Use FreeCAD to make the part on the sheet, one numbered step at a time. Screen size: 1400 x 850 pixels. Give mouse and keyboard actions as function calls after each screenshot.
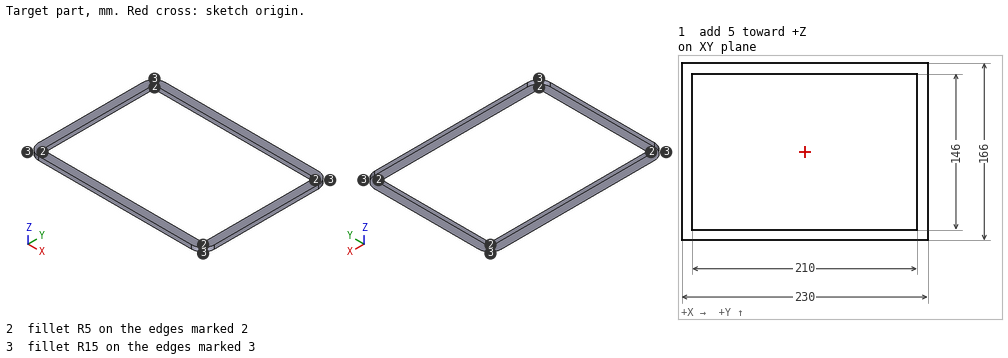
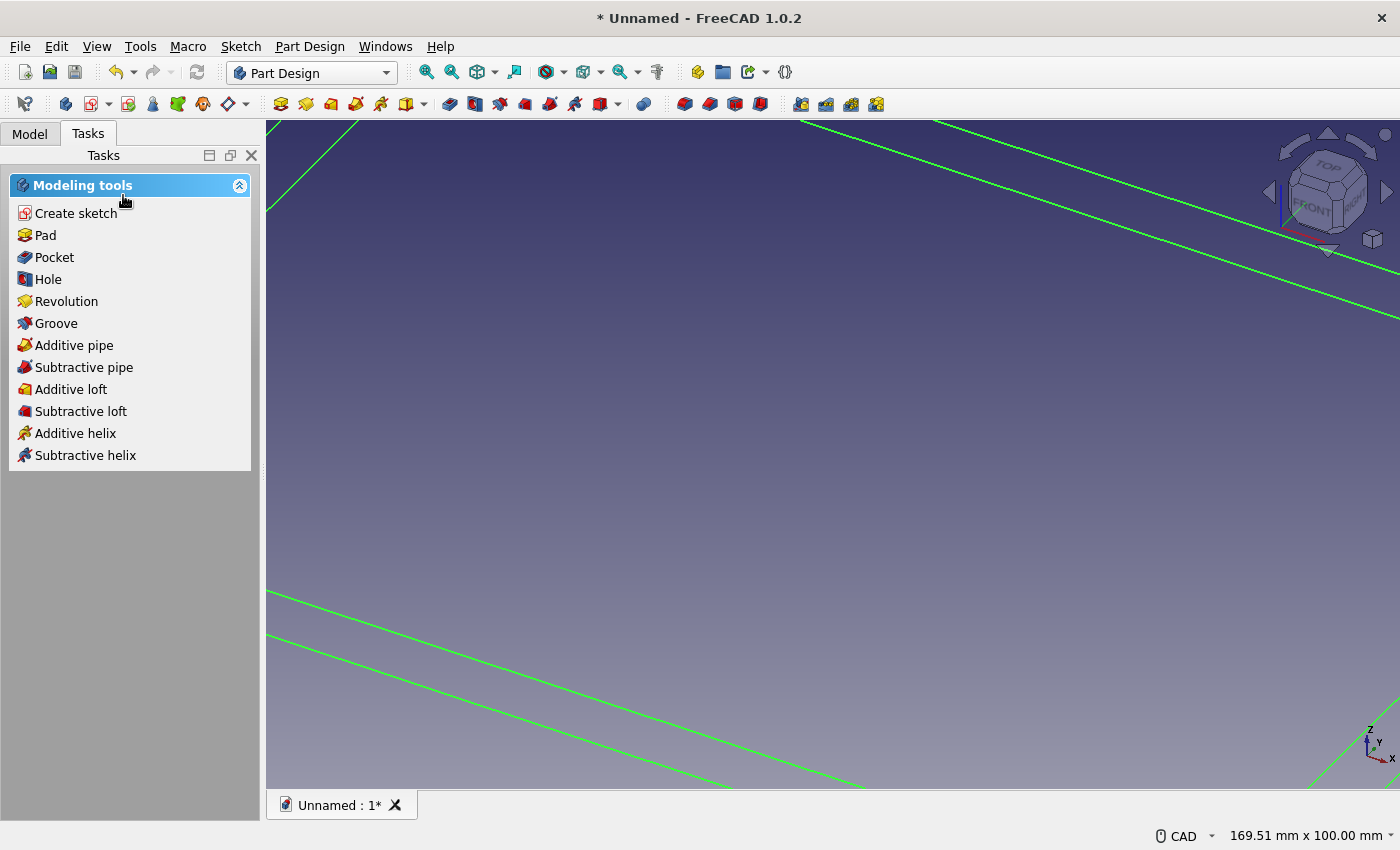
click(281, 104)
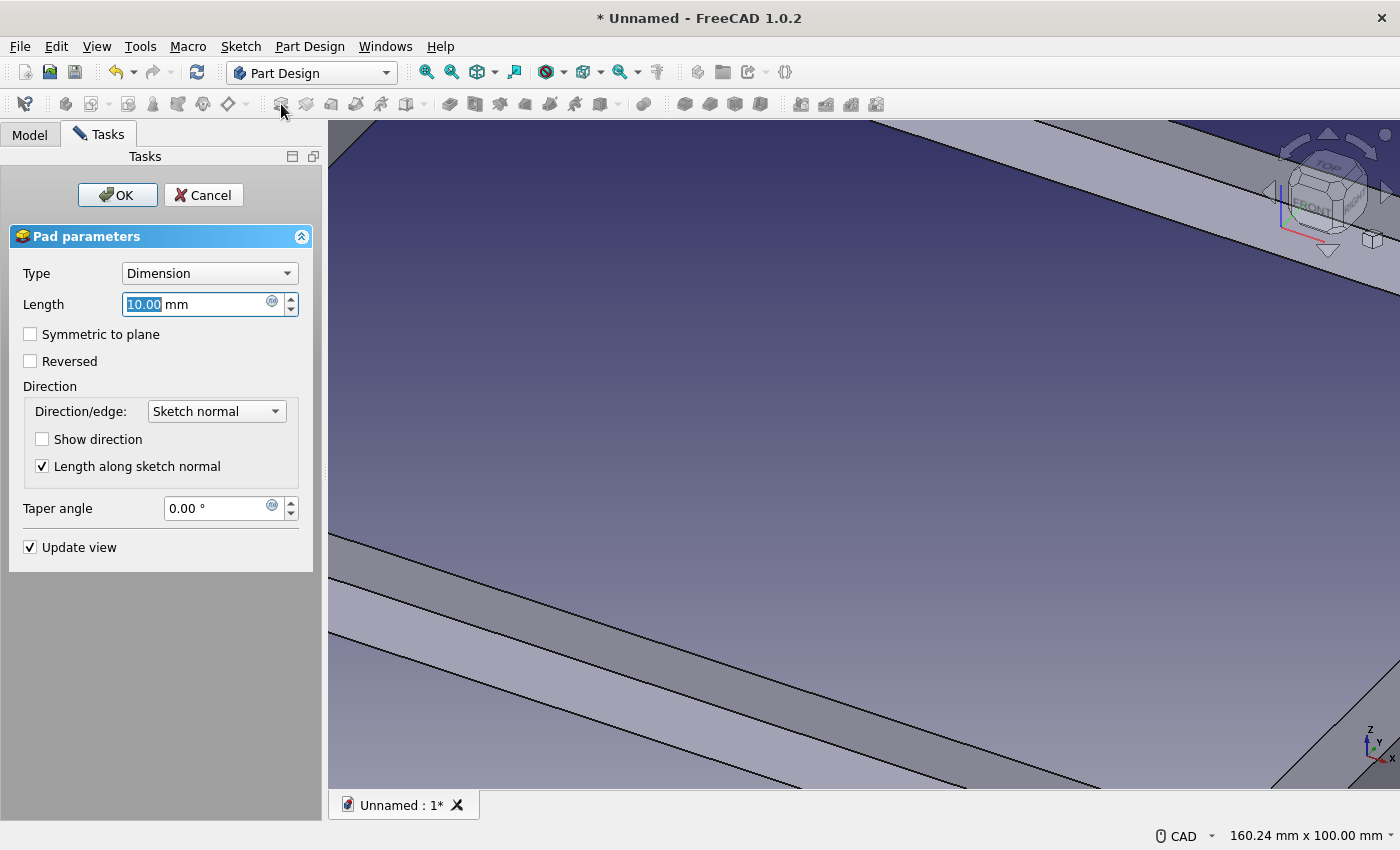
text(5)
key(Tab)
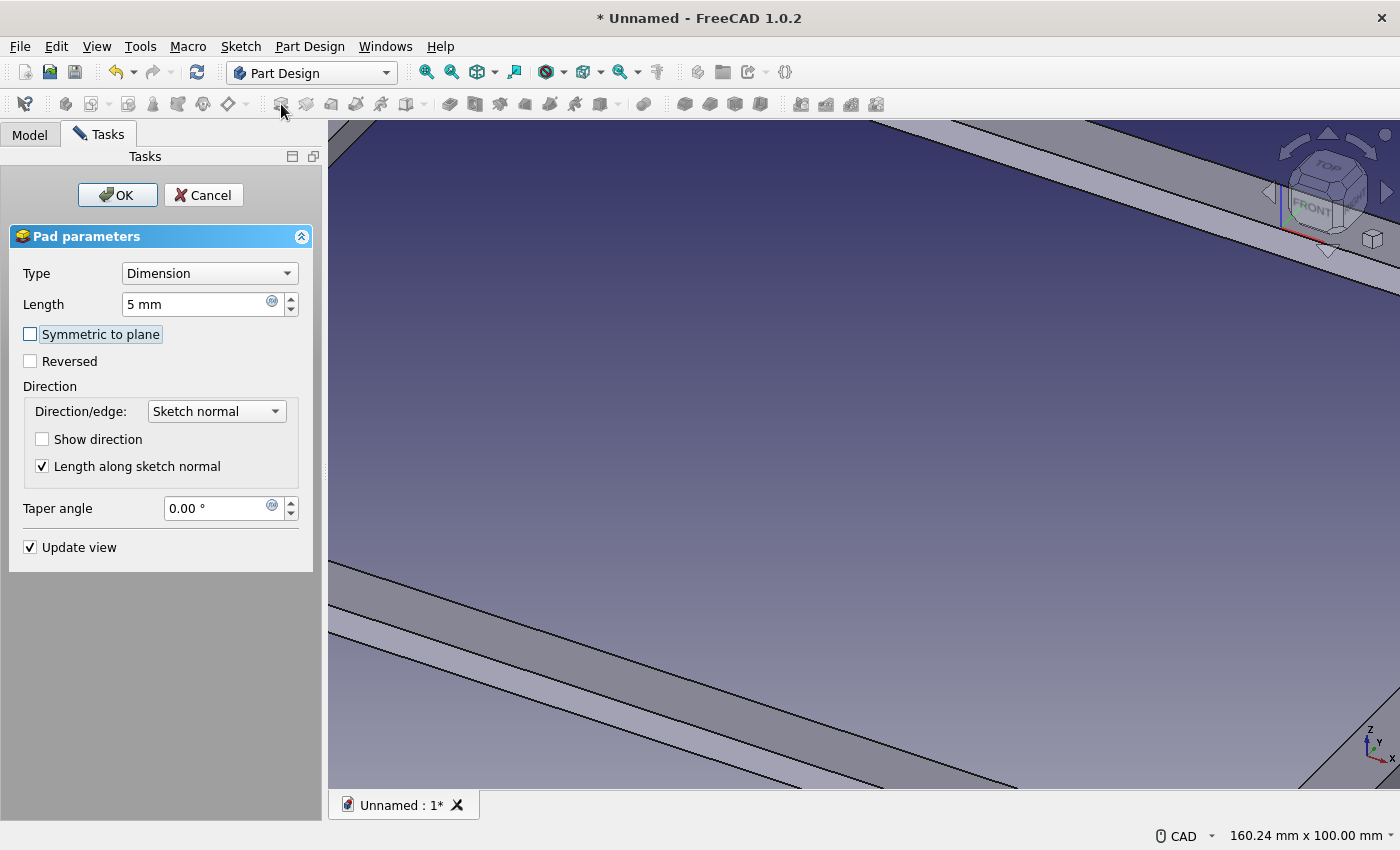
click(118, 195)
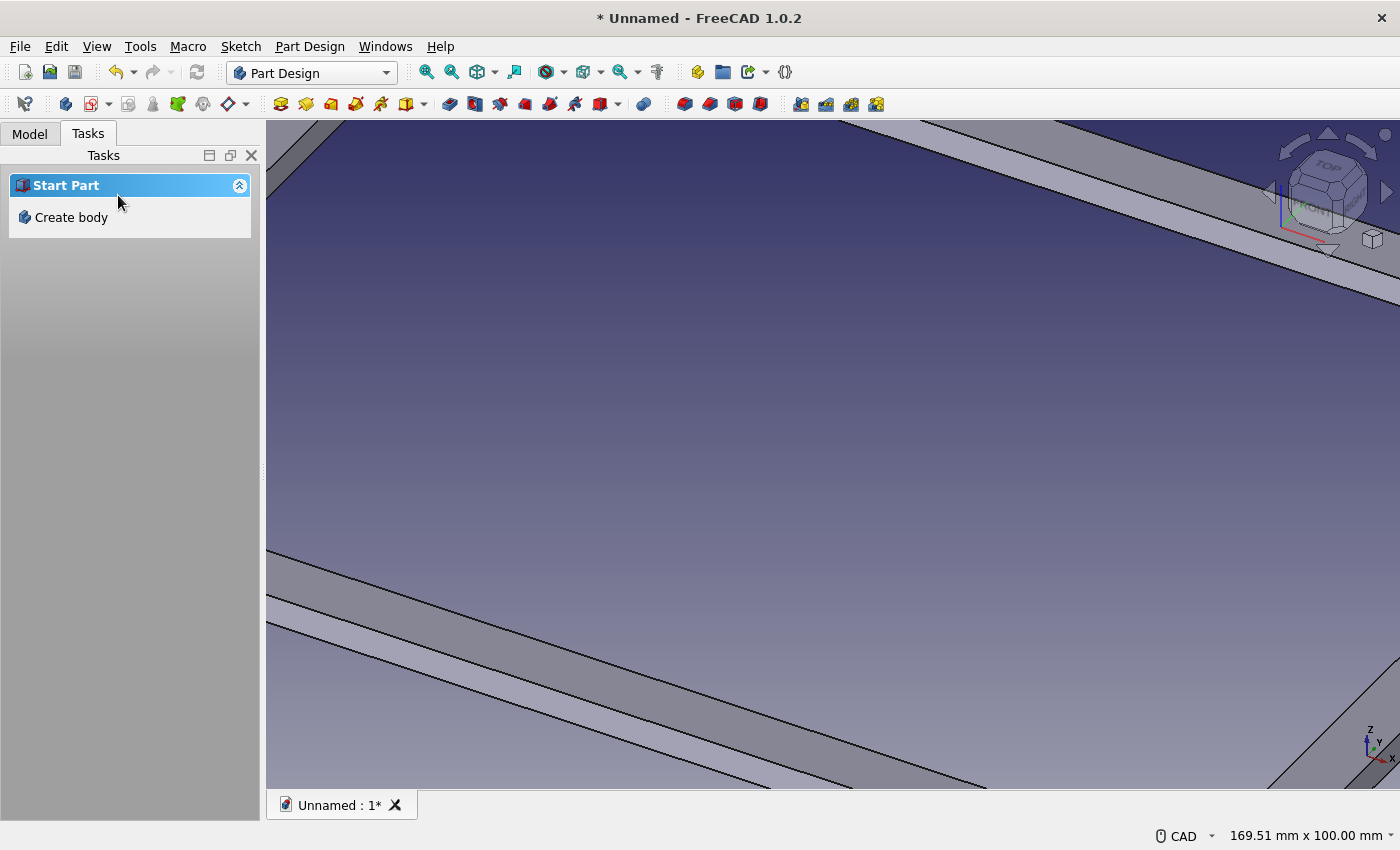
key(v)
key(f)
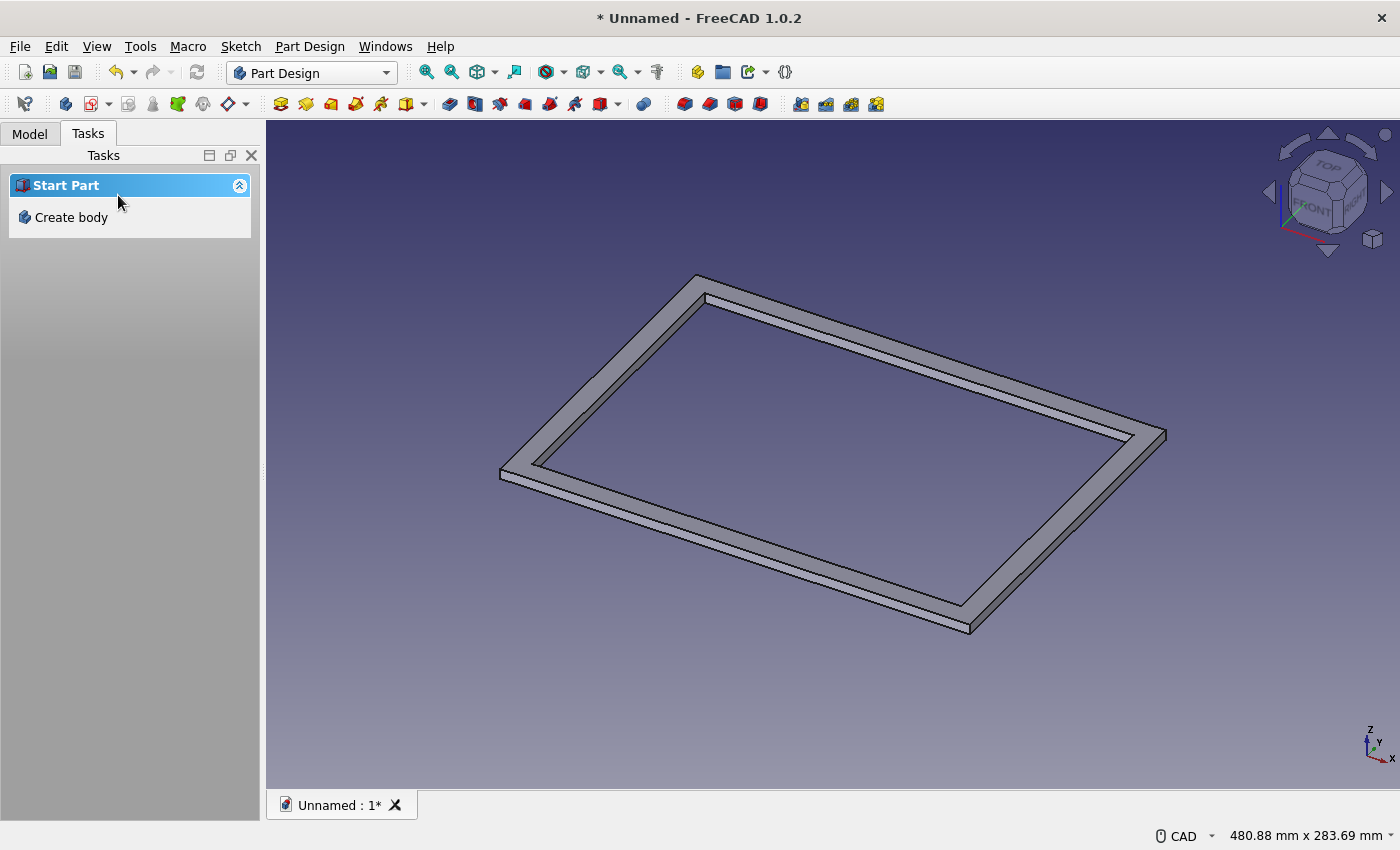
scroll(705, 297, up, 7)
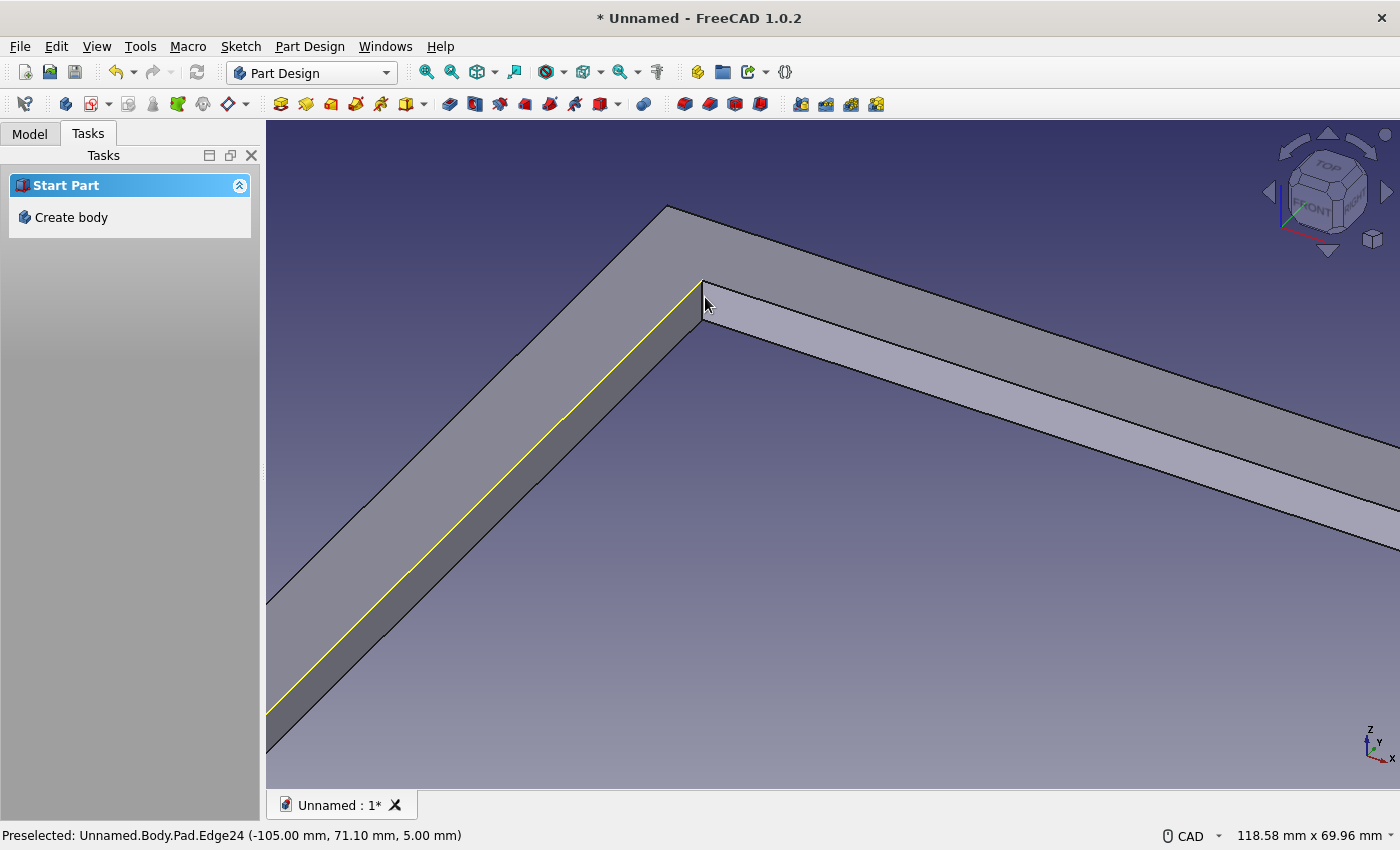
key(v)
key(f)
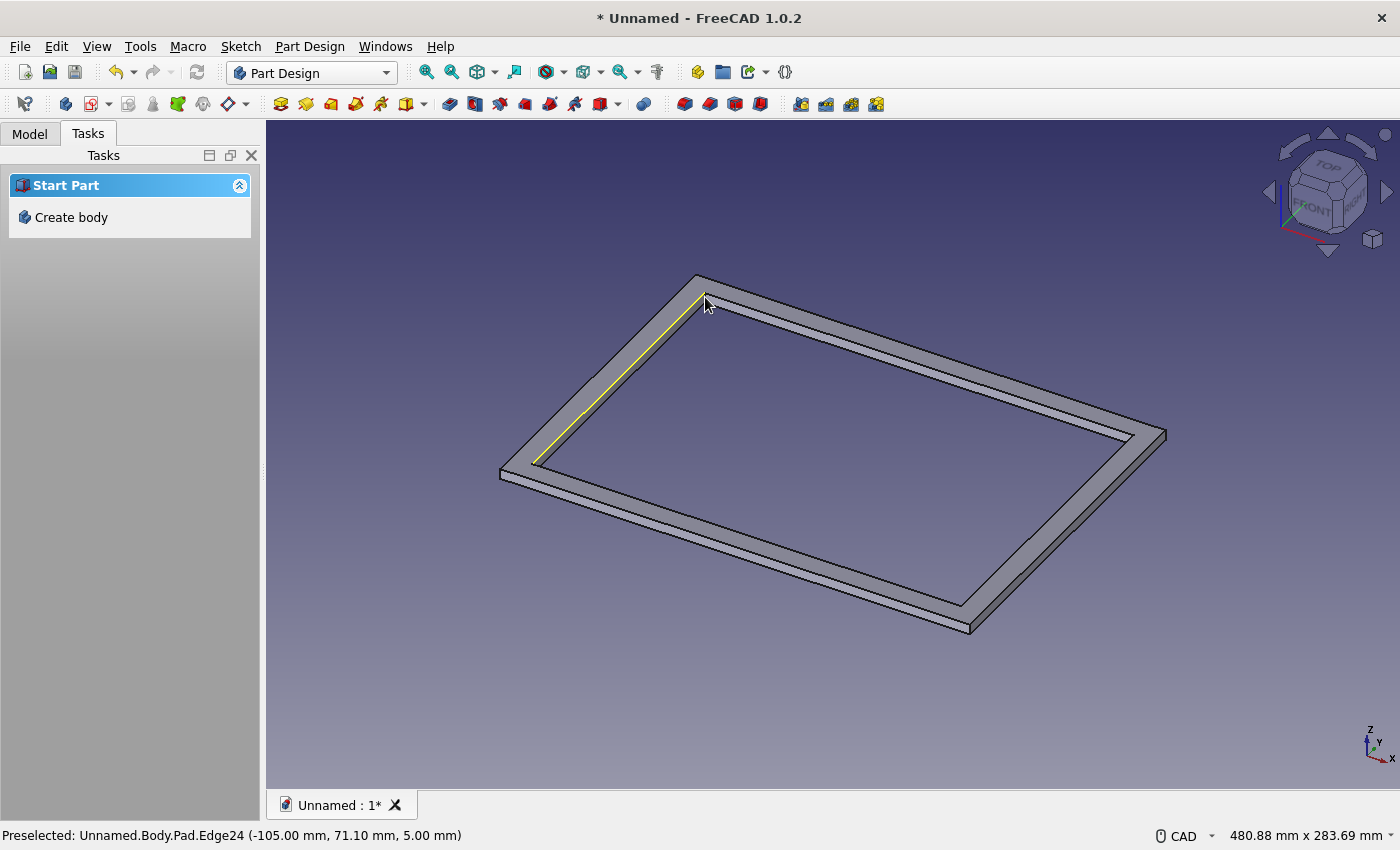
key(0)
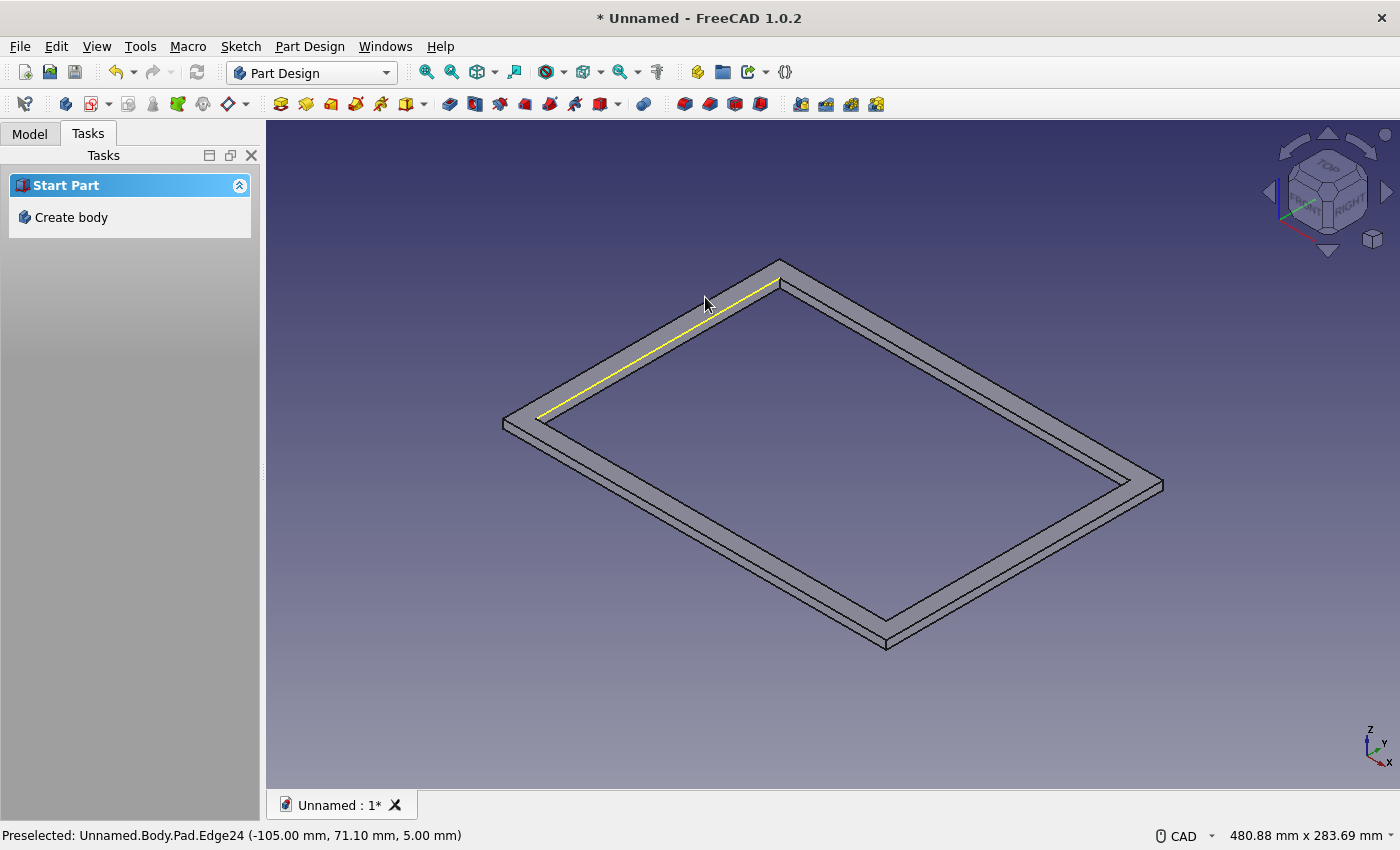
scroll(780, 282, up, 7)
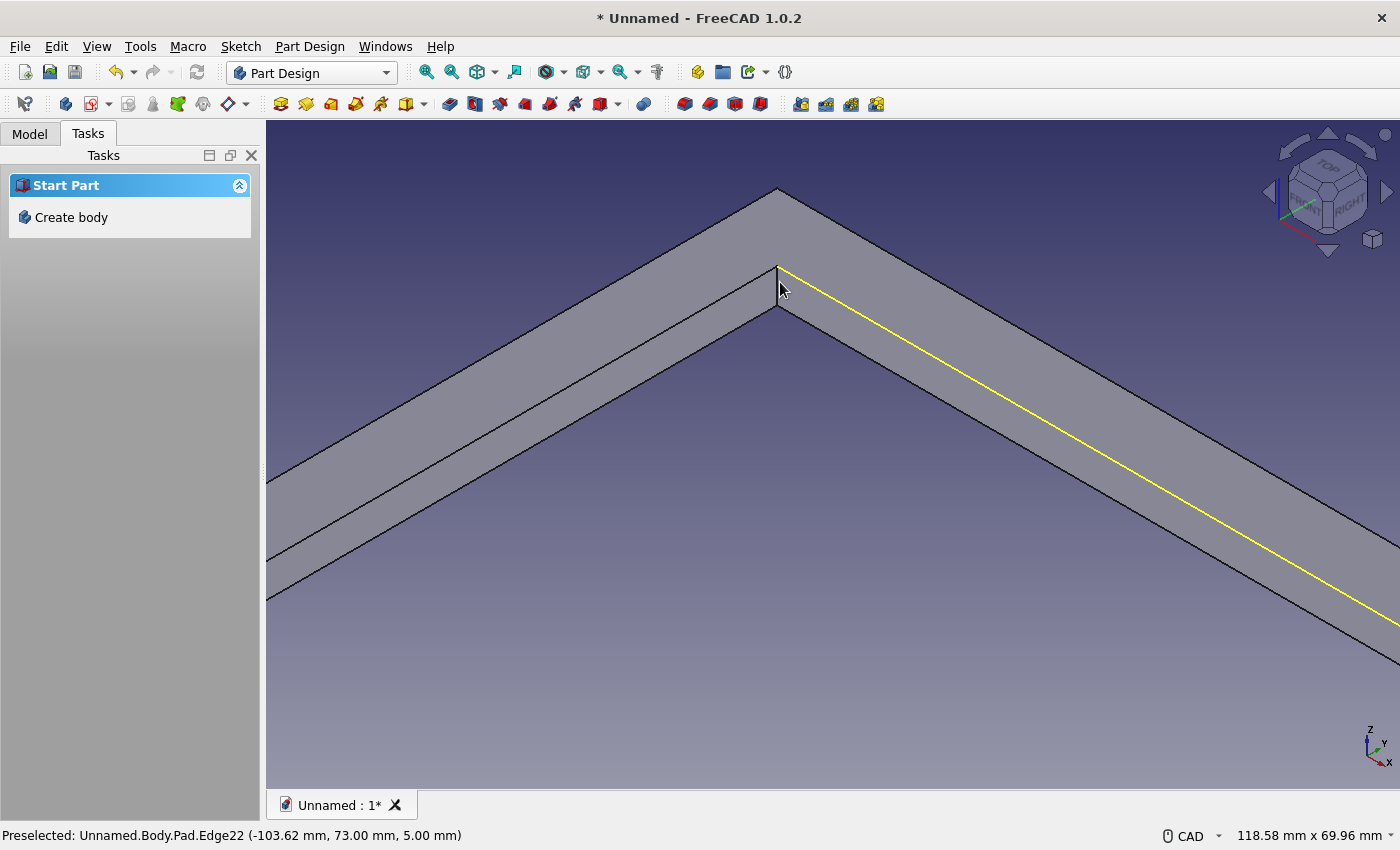
key(v)
key(f)